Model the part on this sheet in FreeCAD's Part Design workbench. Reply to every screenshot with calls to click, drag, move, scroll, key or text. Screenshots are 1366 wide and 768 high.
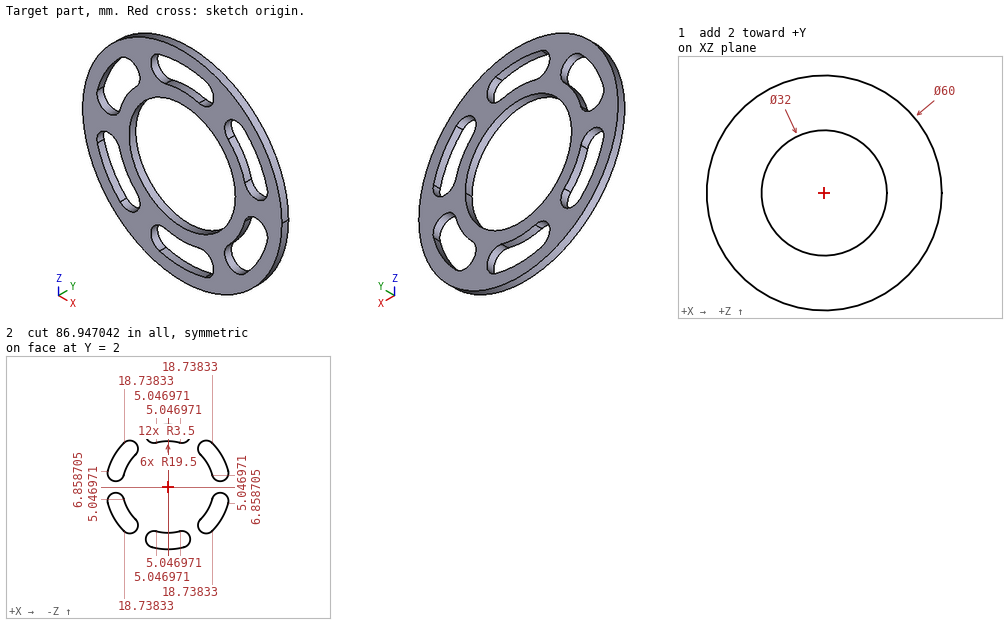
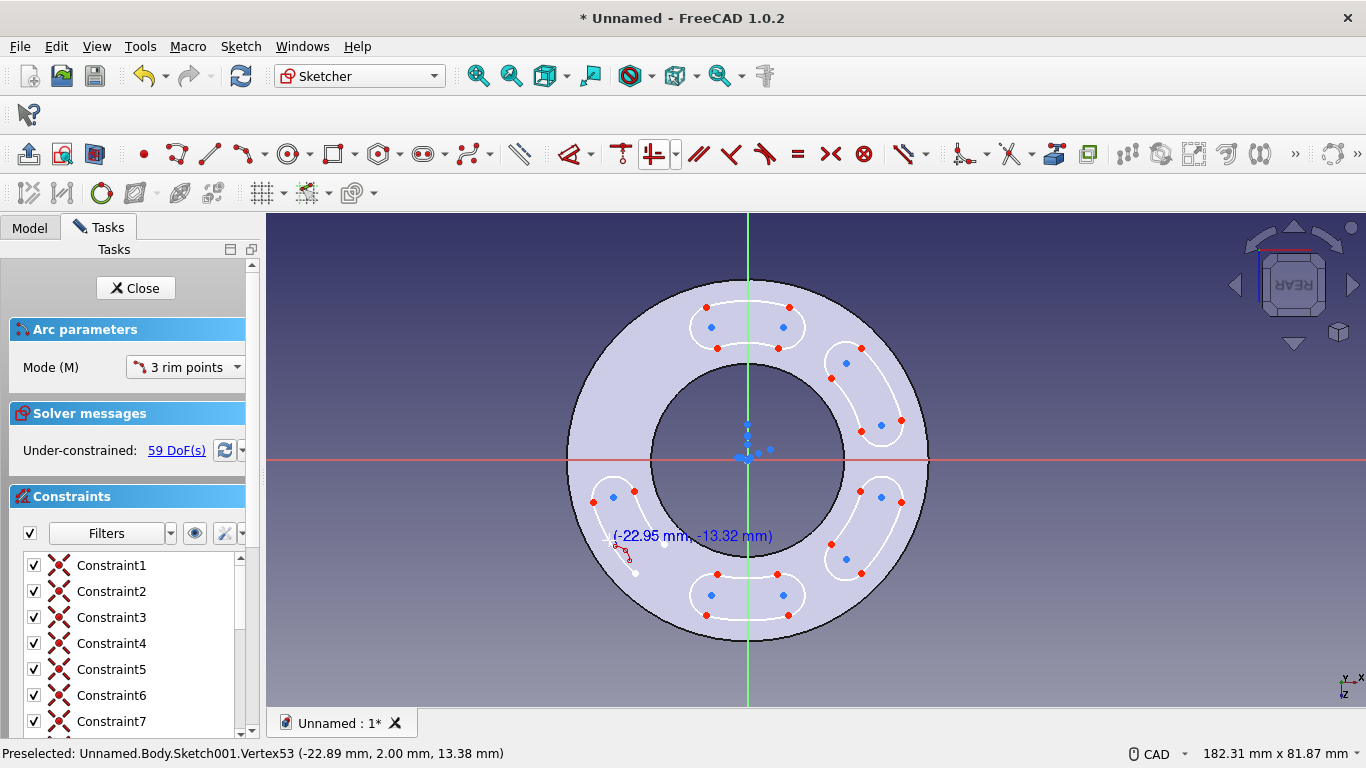
click(635, 574)
click(664, 545)
click(664, 573)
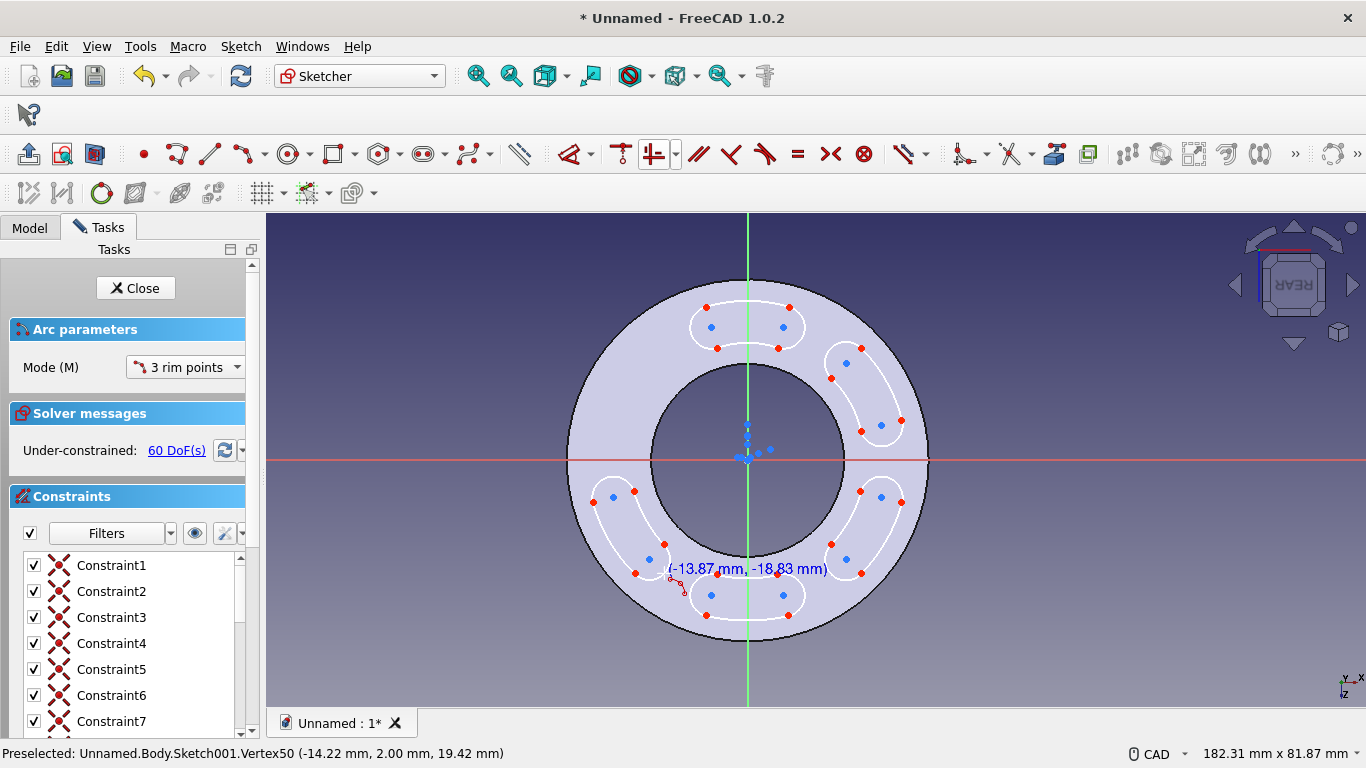
click(664, 377)
click(635, 347)
click(664, 347)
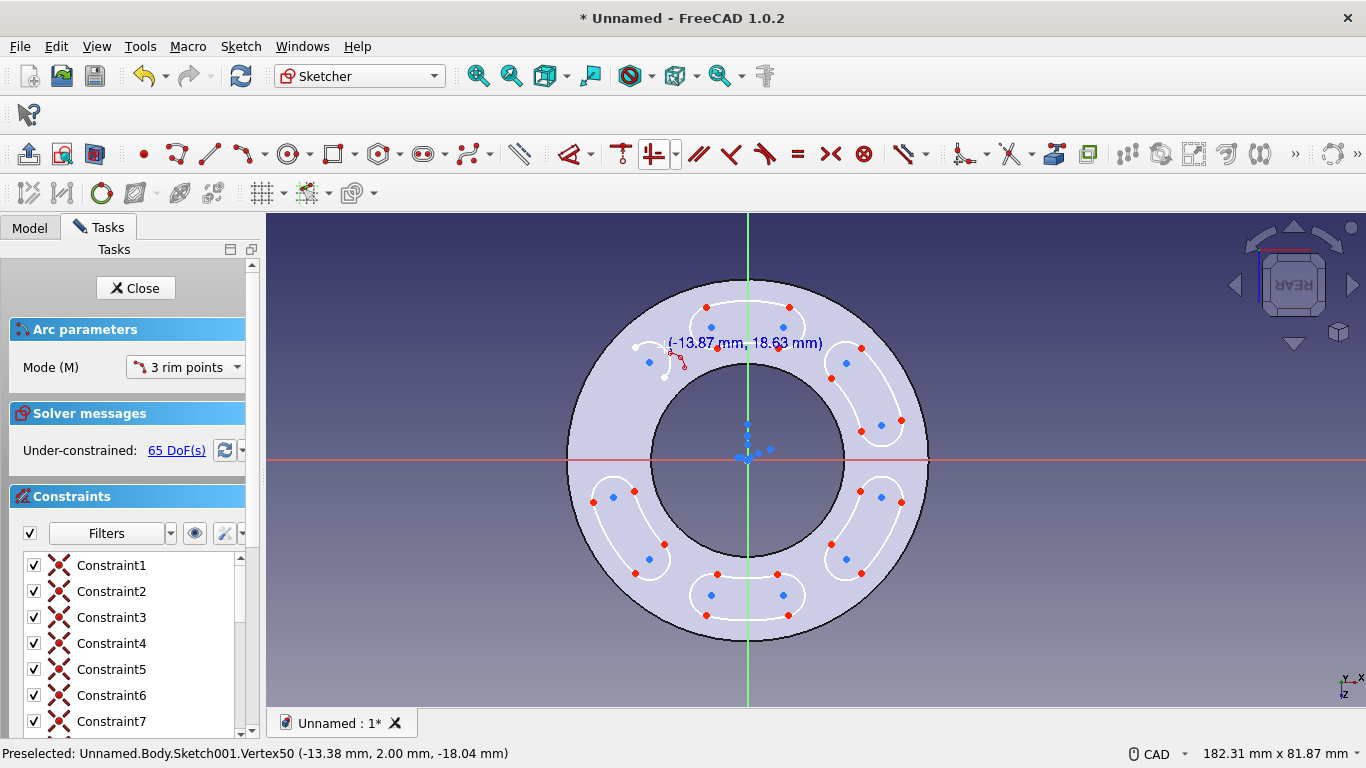
click(635, 348)
click(593, 419)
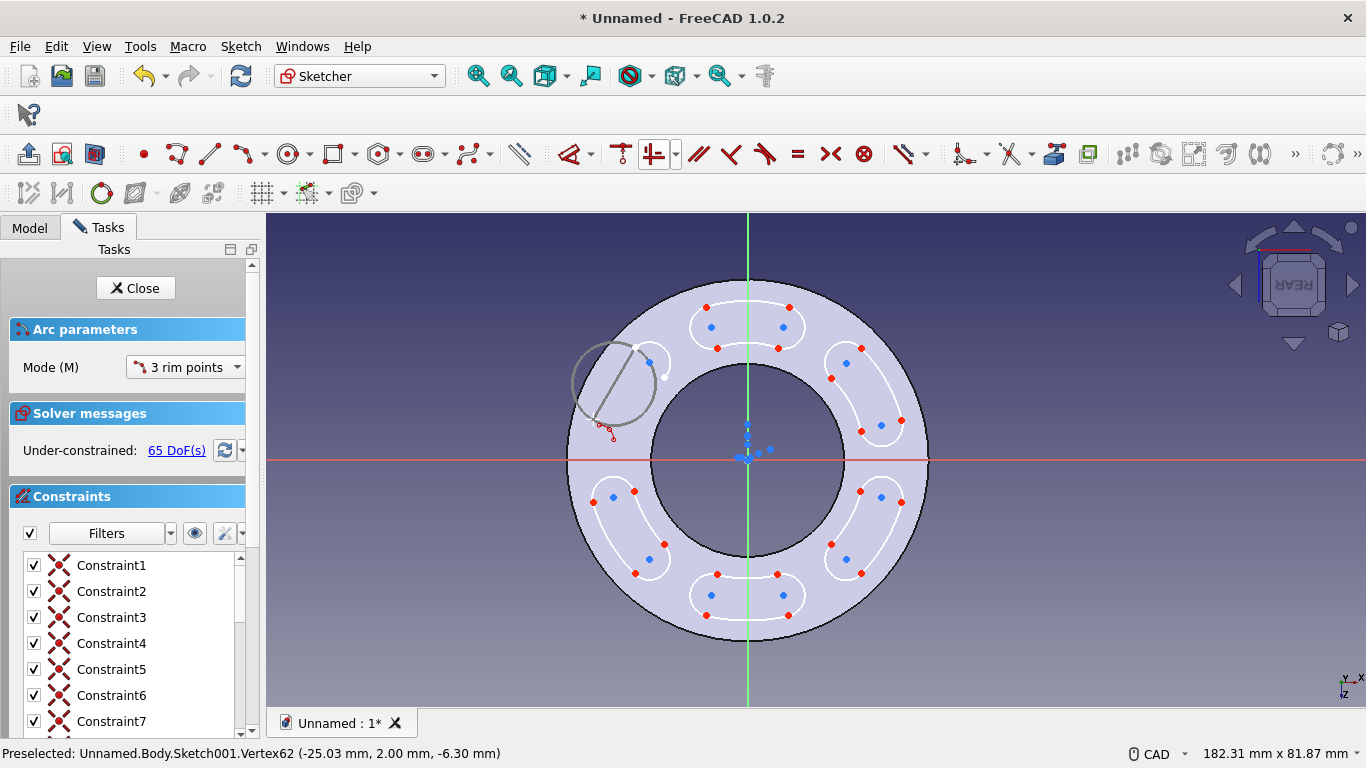
scroll(609, 380, up, 6)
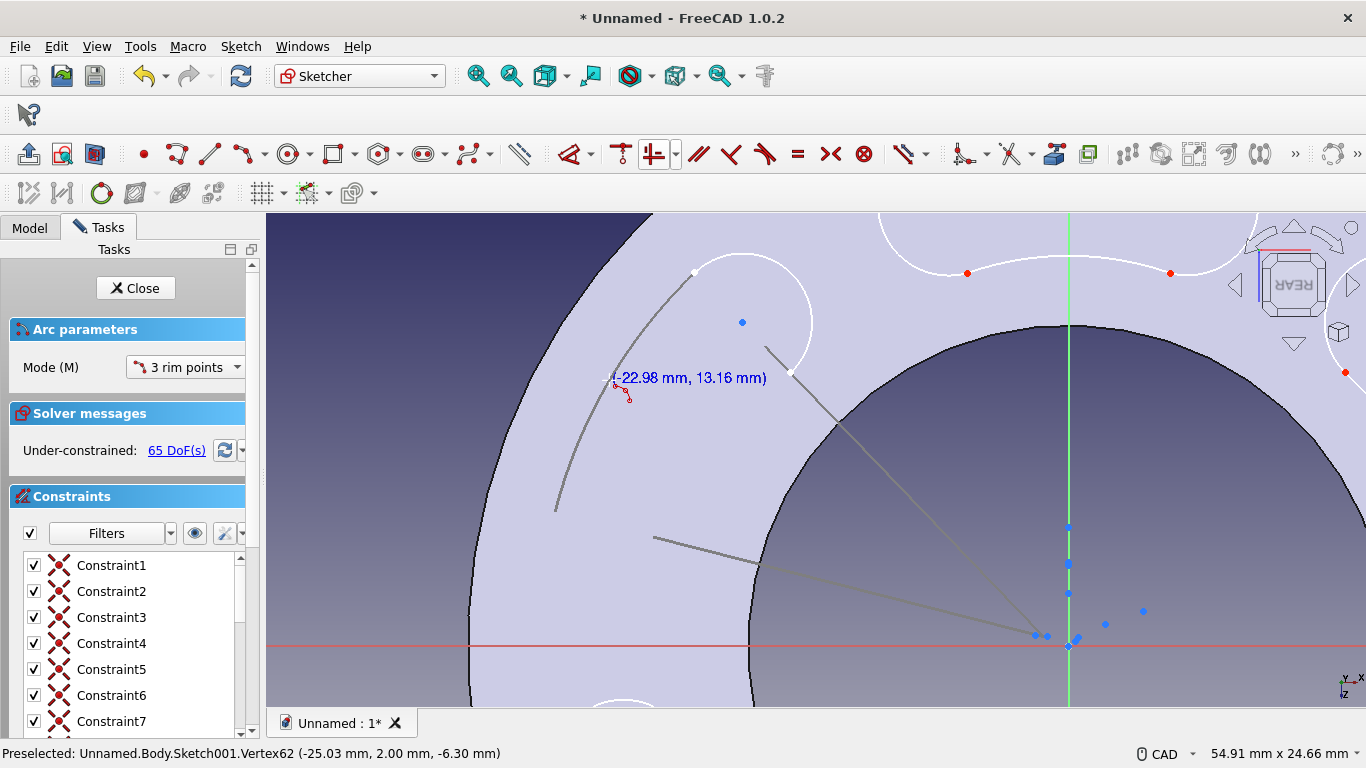
click(609, 381)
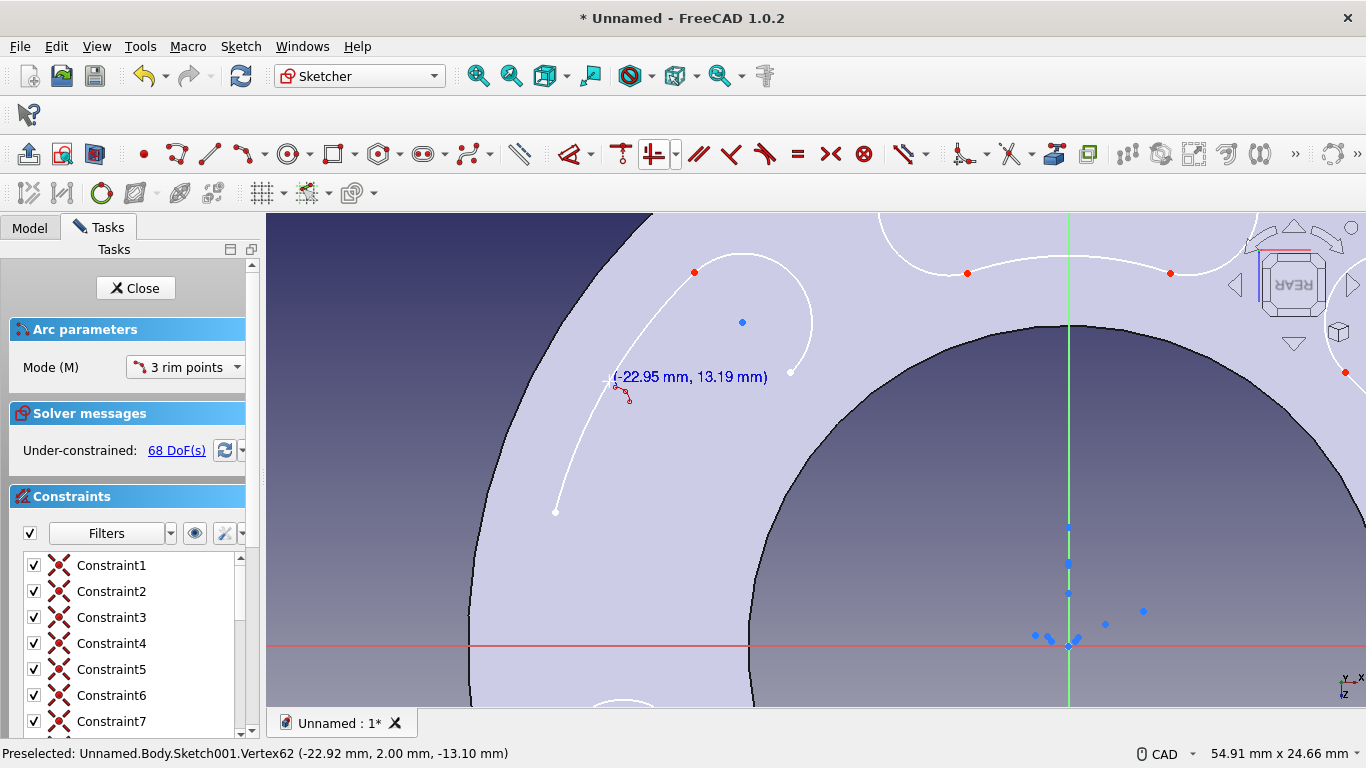
scroll(609, 380, down, 6)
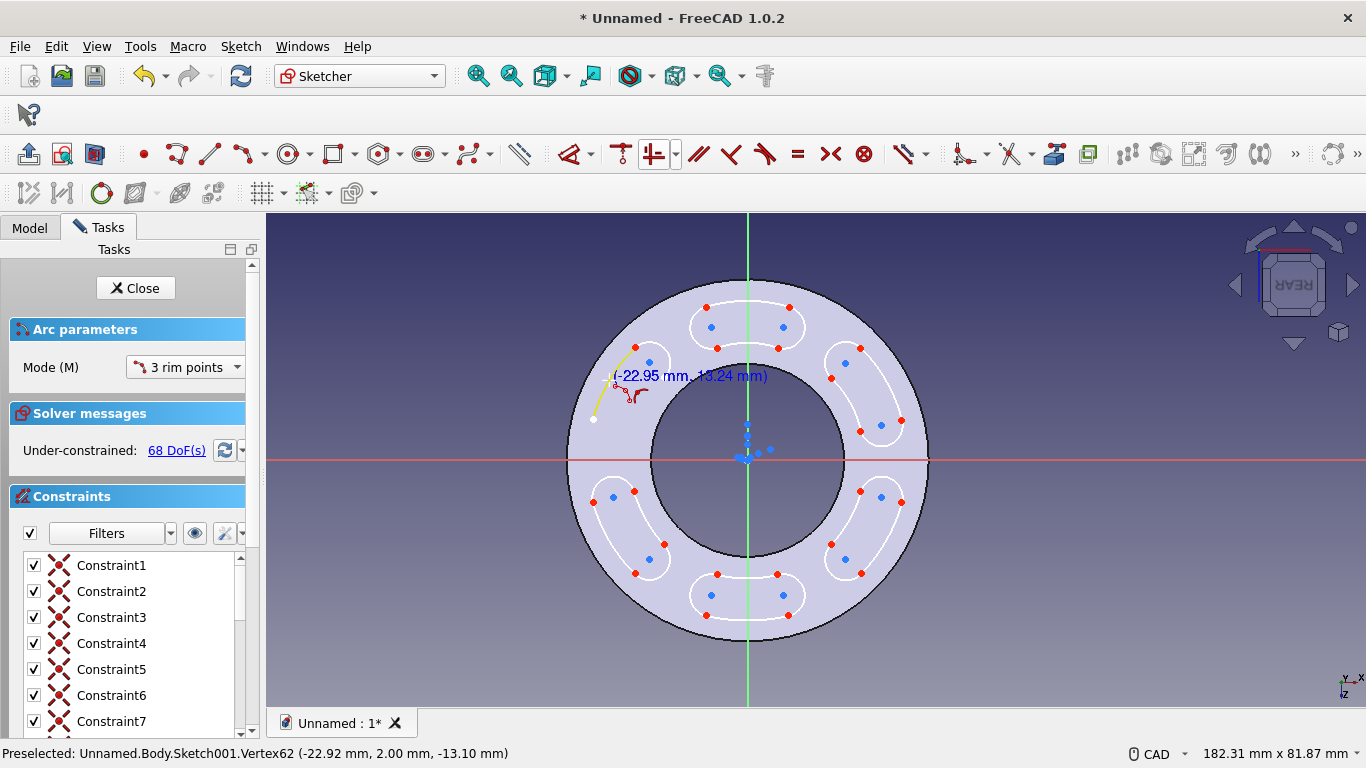
click(593, 420)
click(634, 430)
click(602, 442)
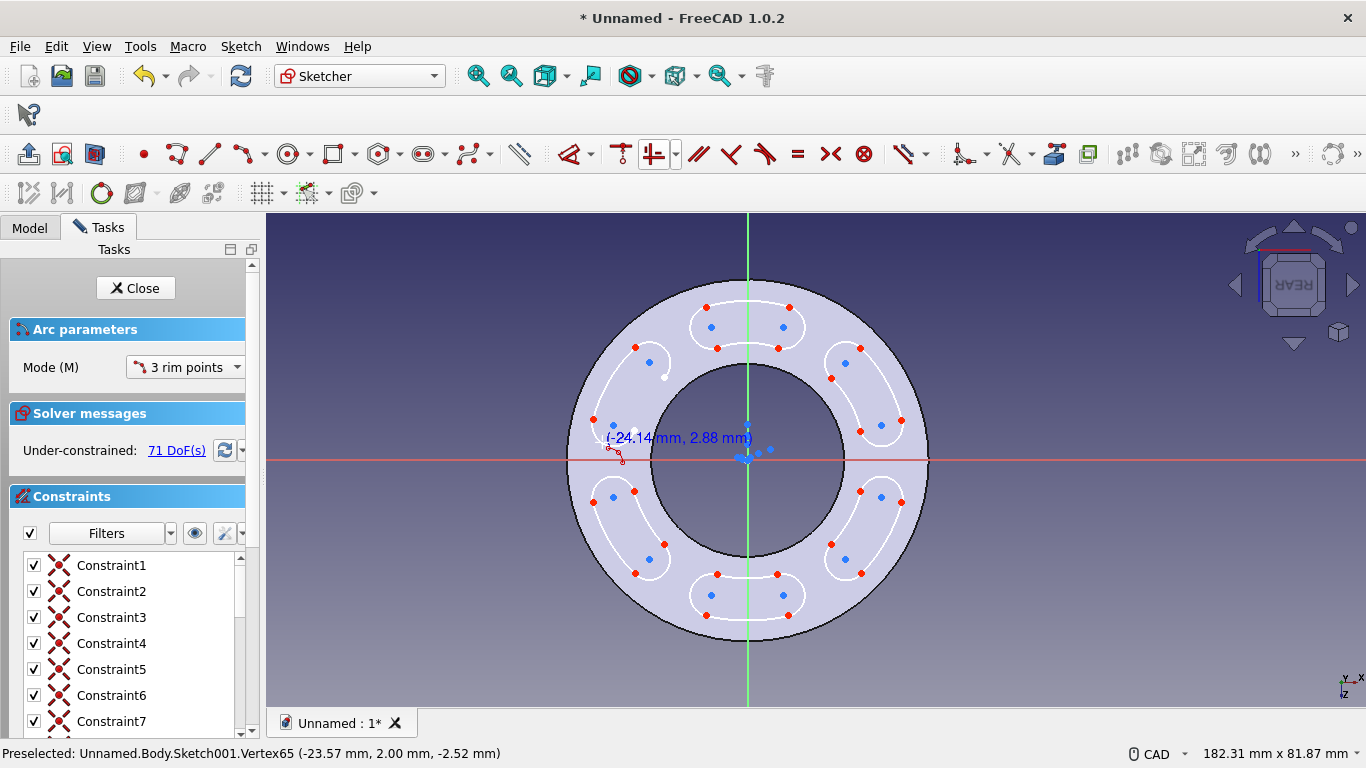
click(634, 431)
click(664, 378)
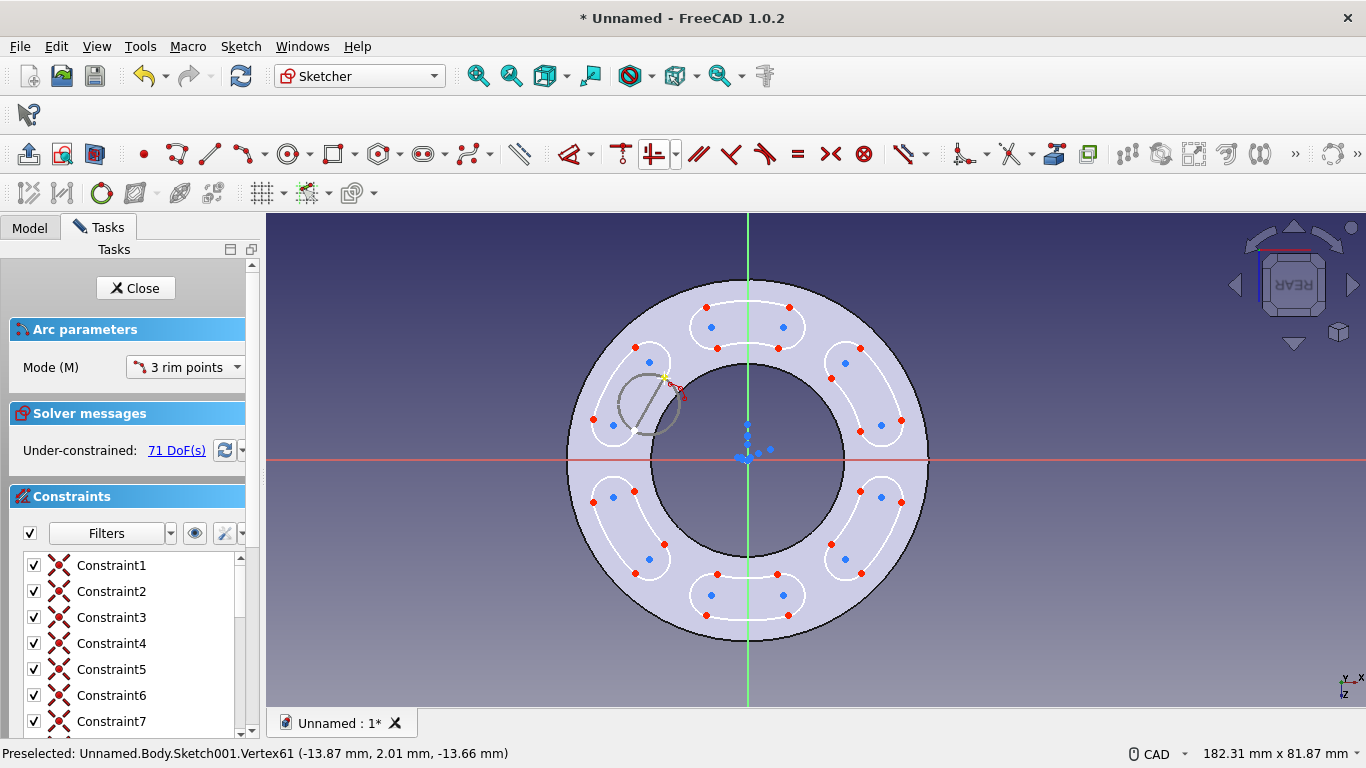
scroll(646, 402, up, 7)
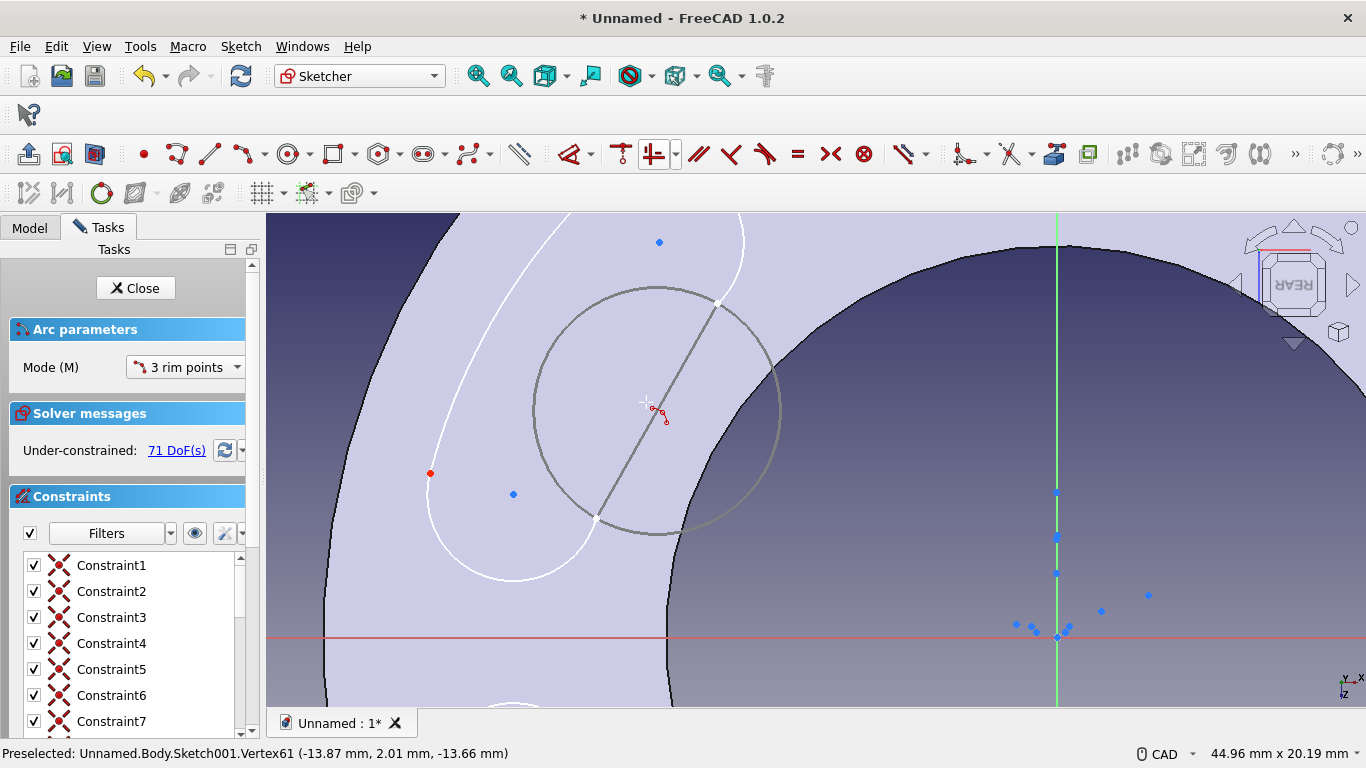
click(644, 399)
key(Escape)